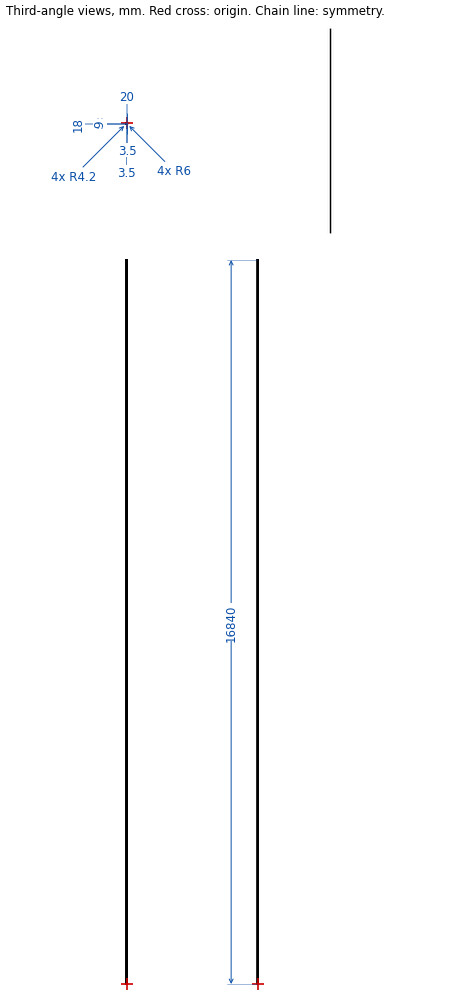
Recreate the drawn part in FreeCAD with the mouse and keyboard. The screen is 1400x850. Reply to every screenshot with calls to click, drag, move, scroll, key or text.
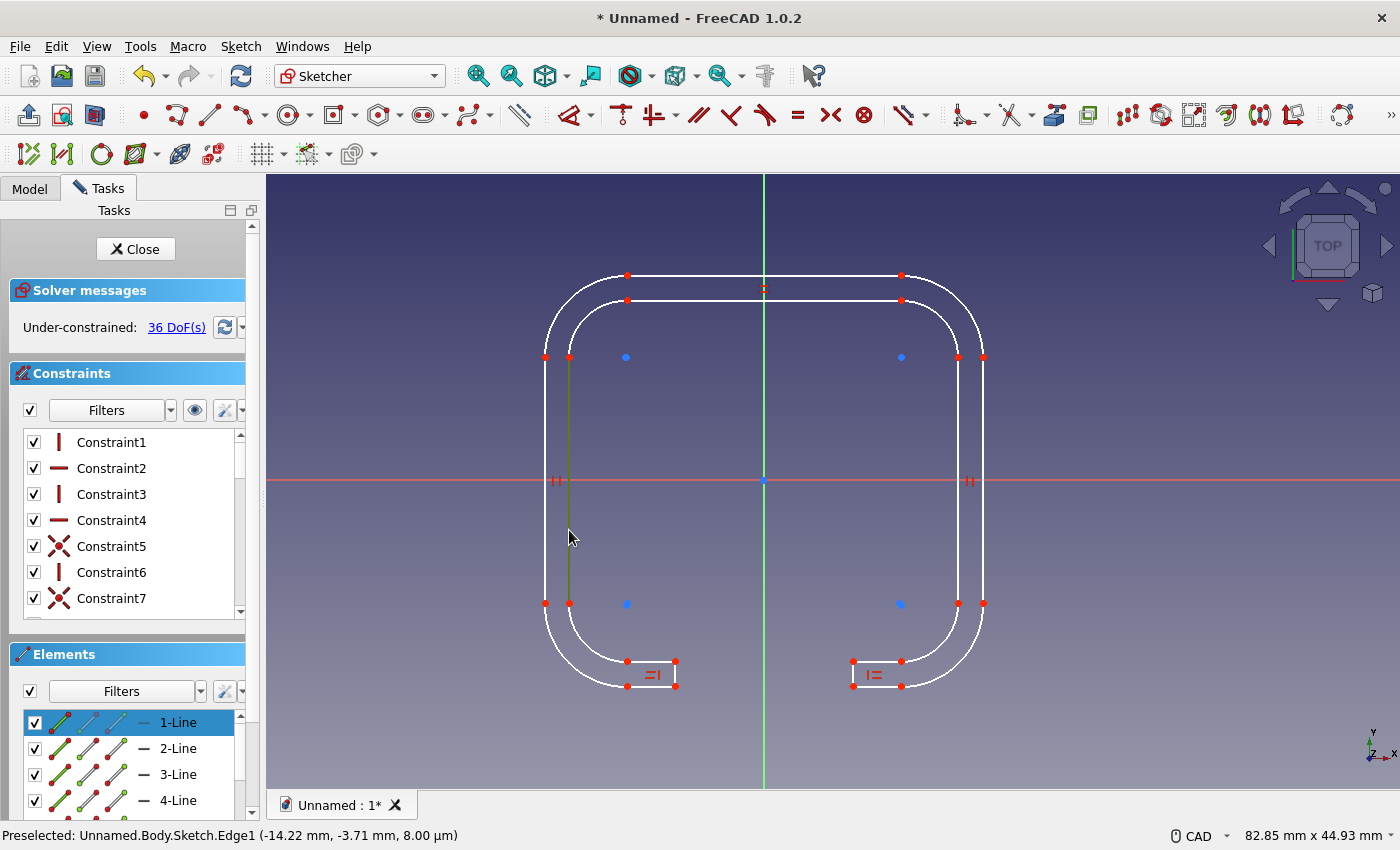
click(601, 307)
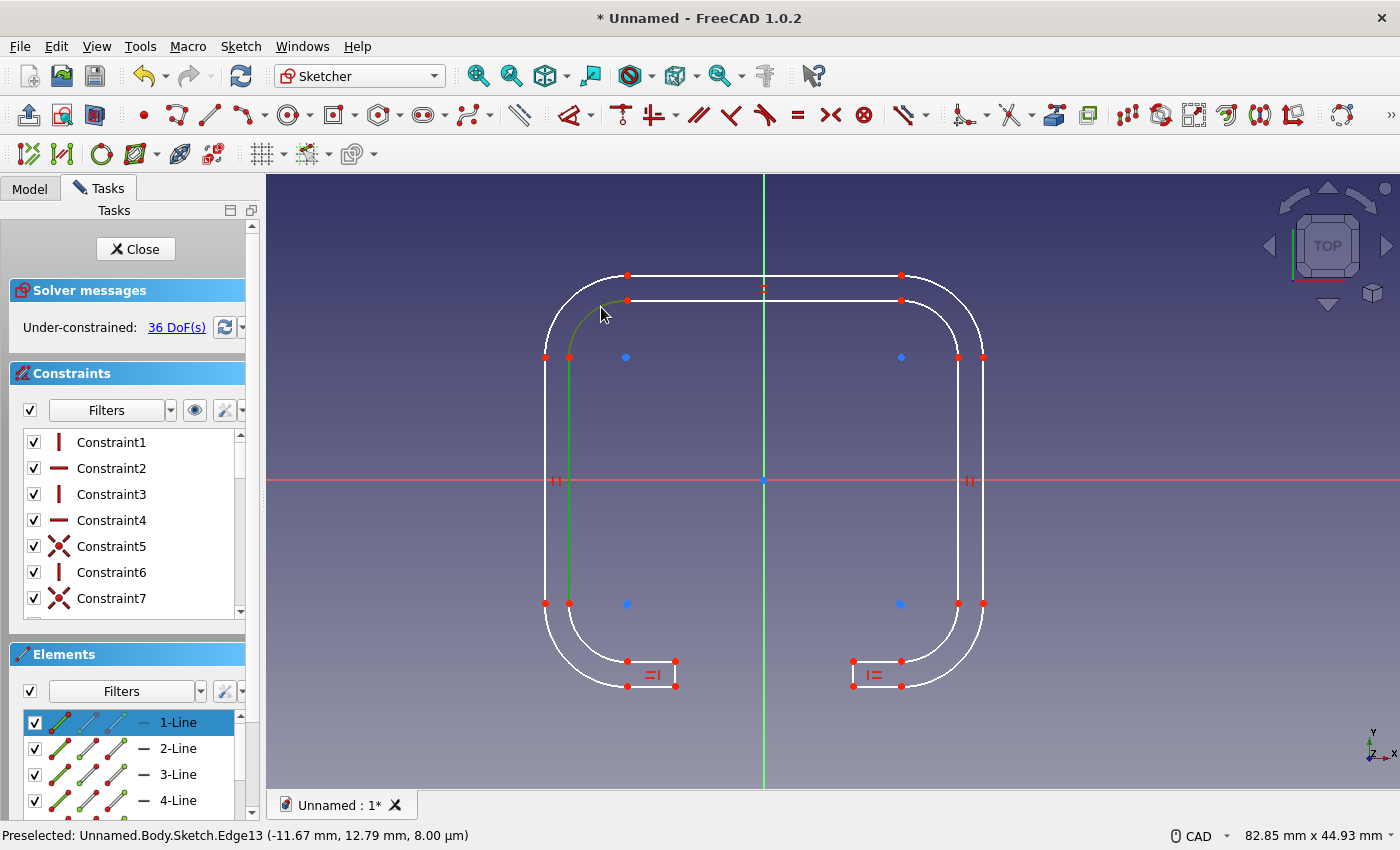
click(765, 116)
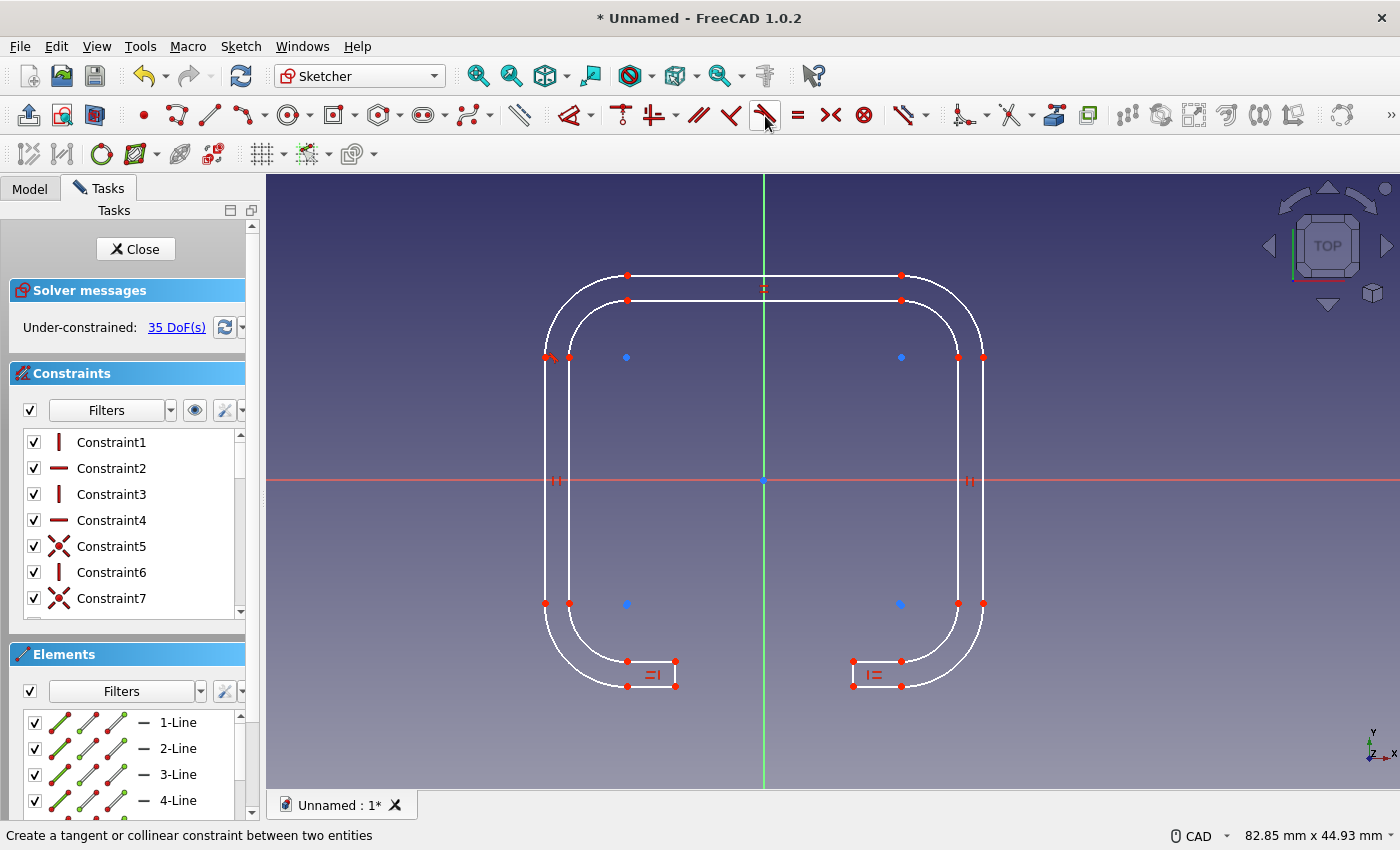
click(569, 530)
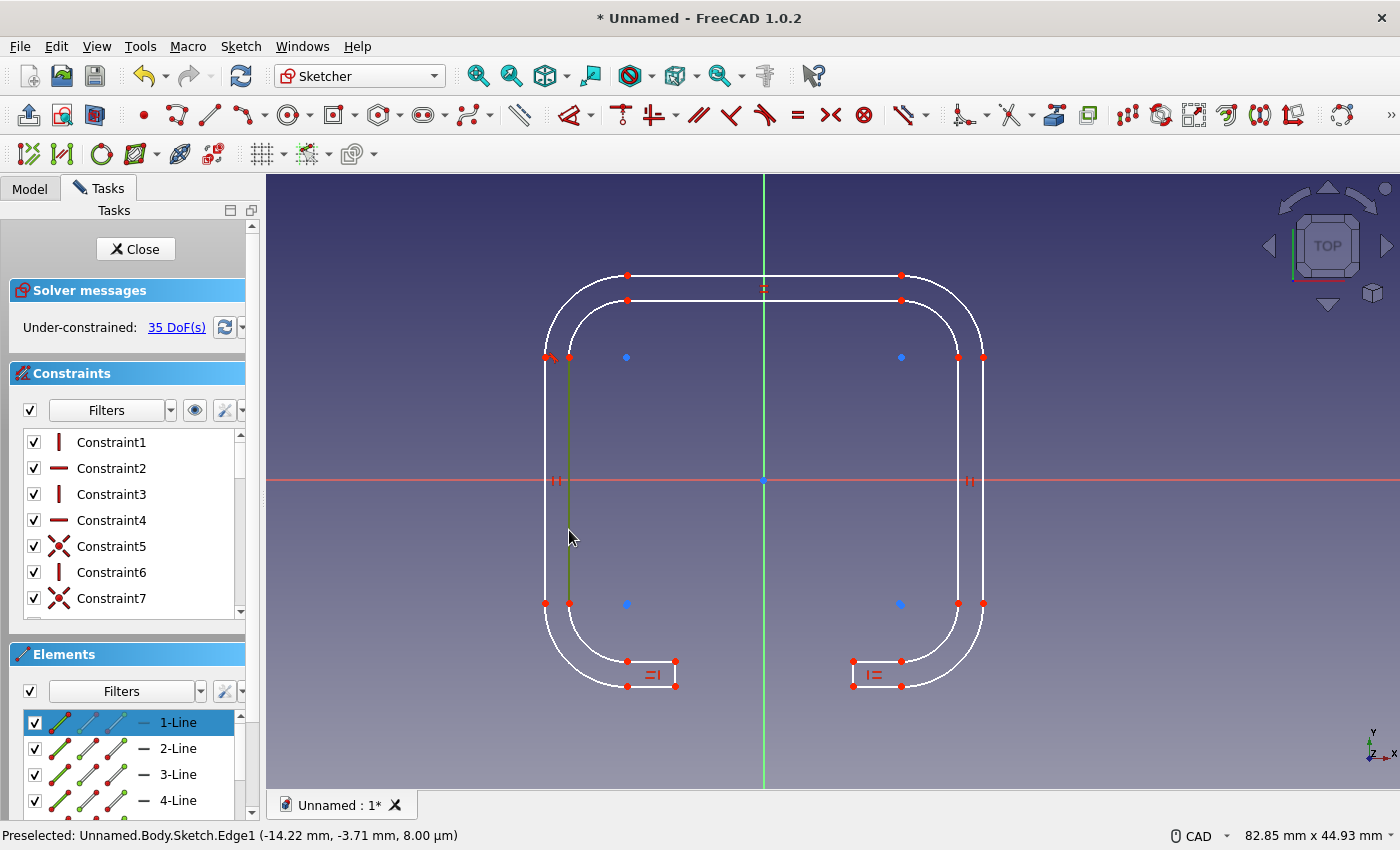
click(575, 630)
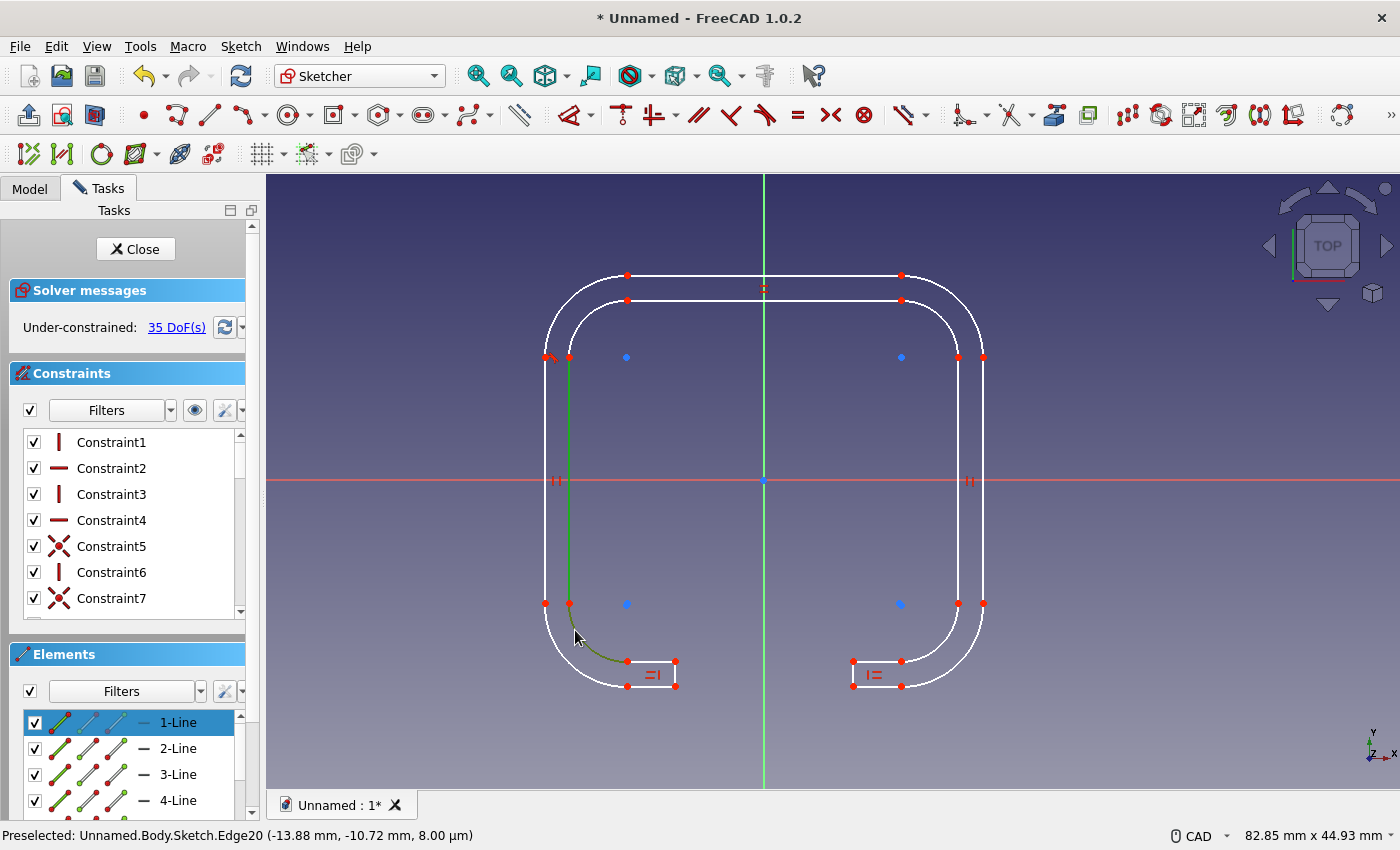
click(765, 116)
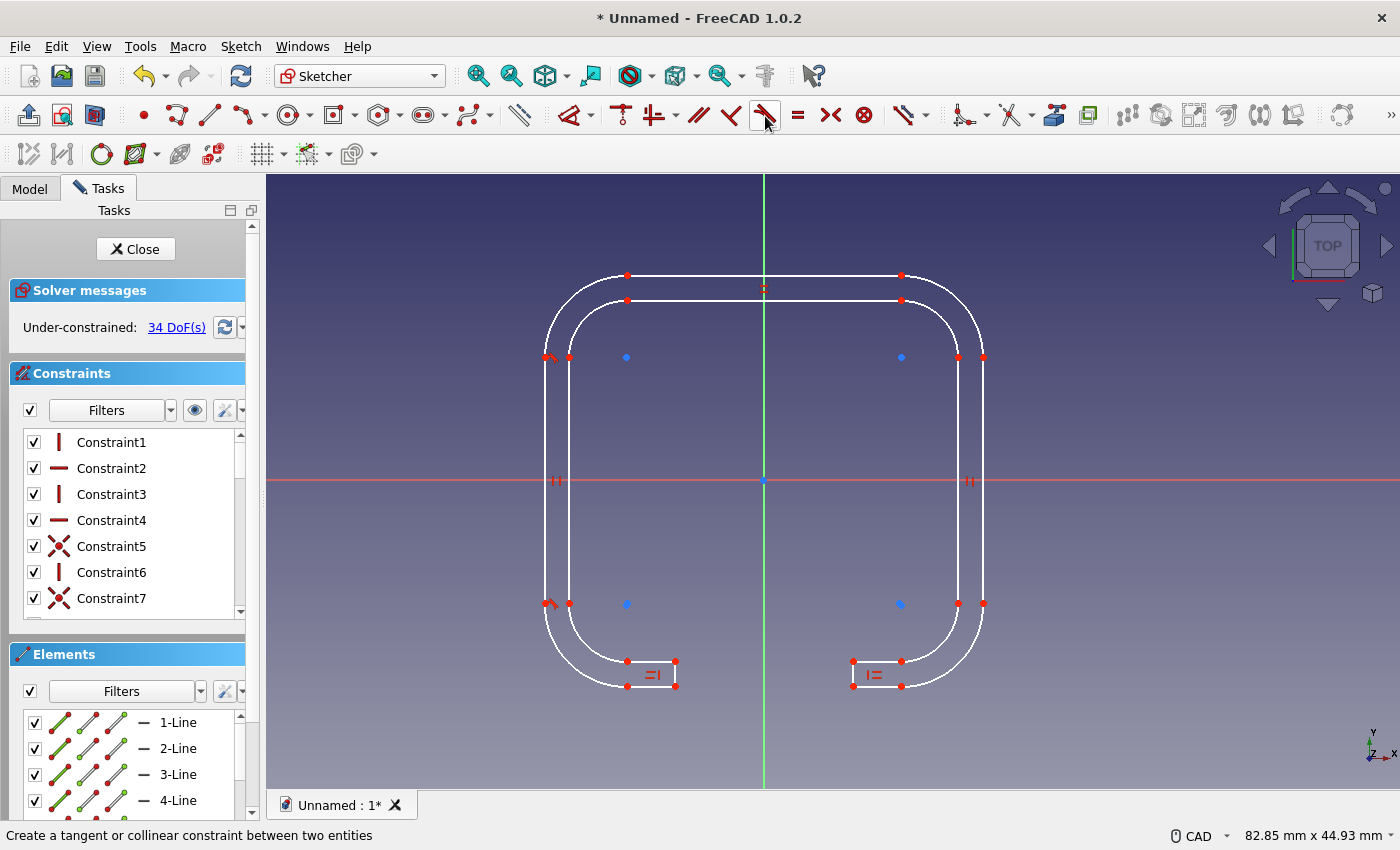
click(709, 301)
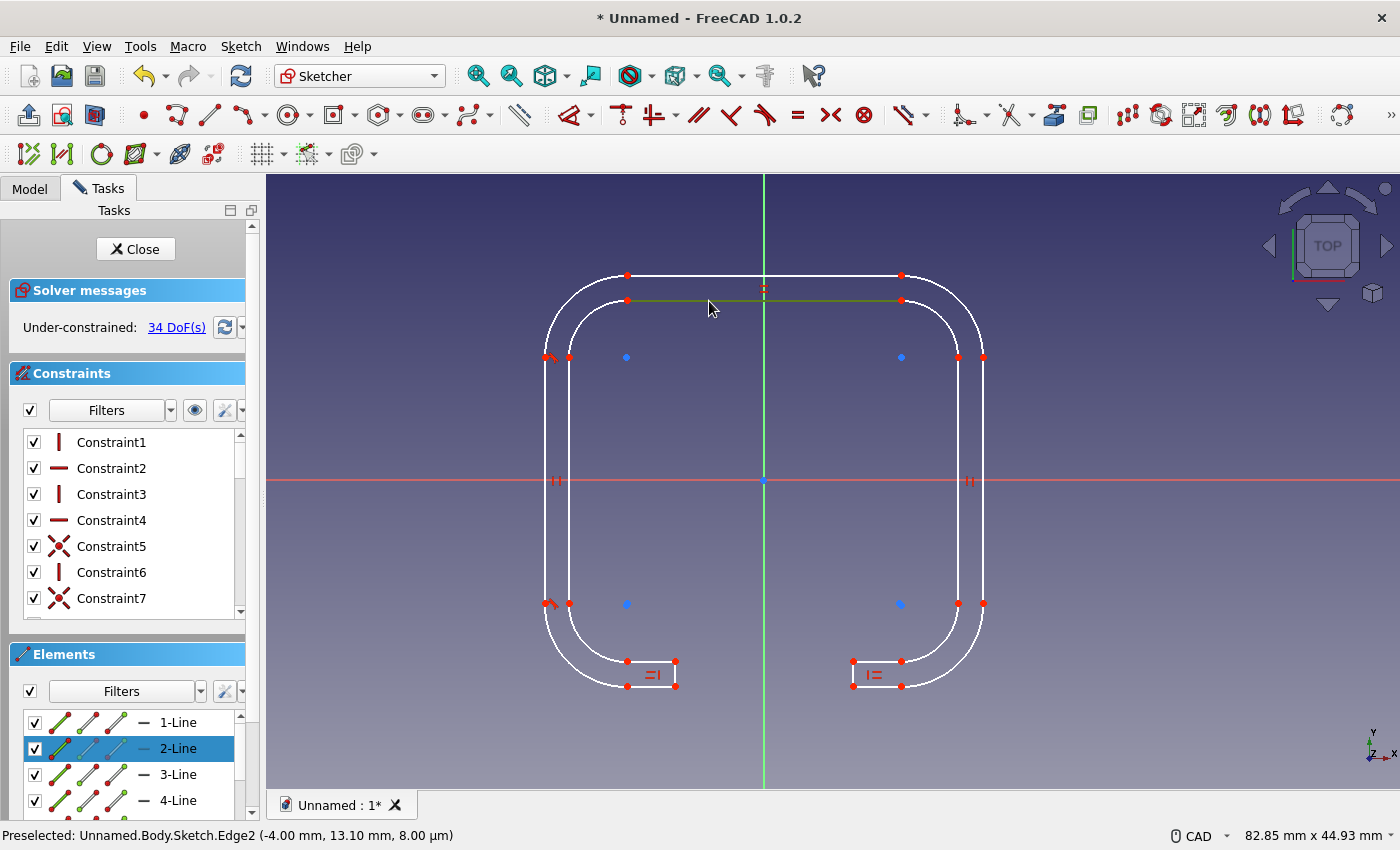
click(601, 307)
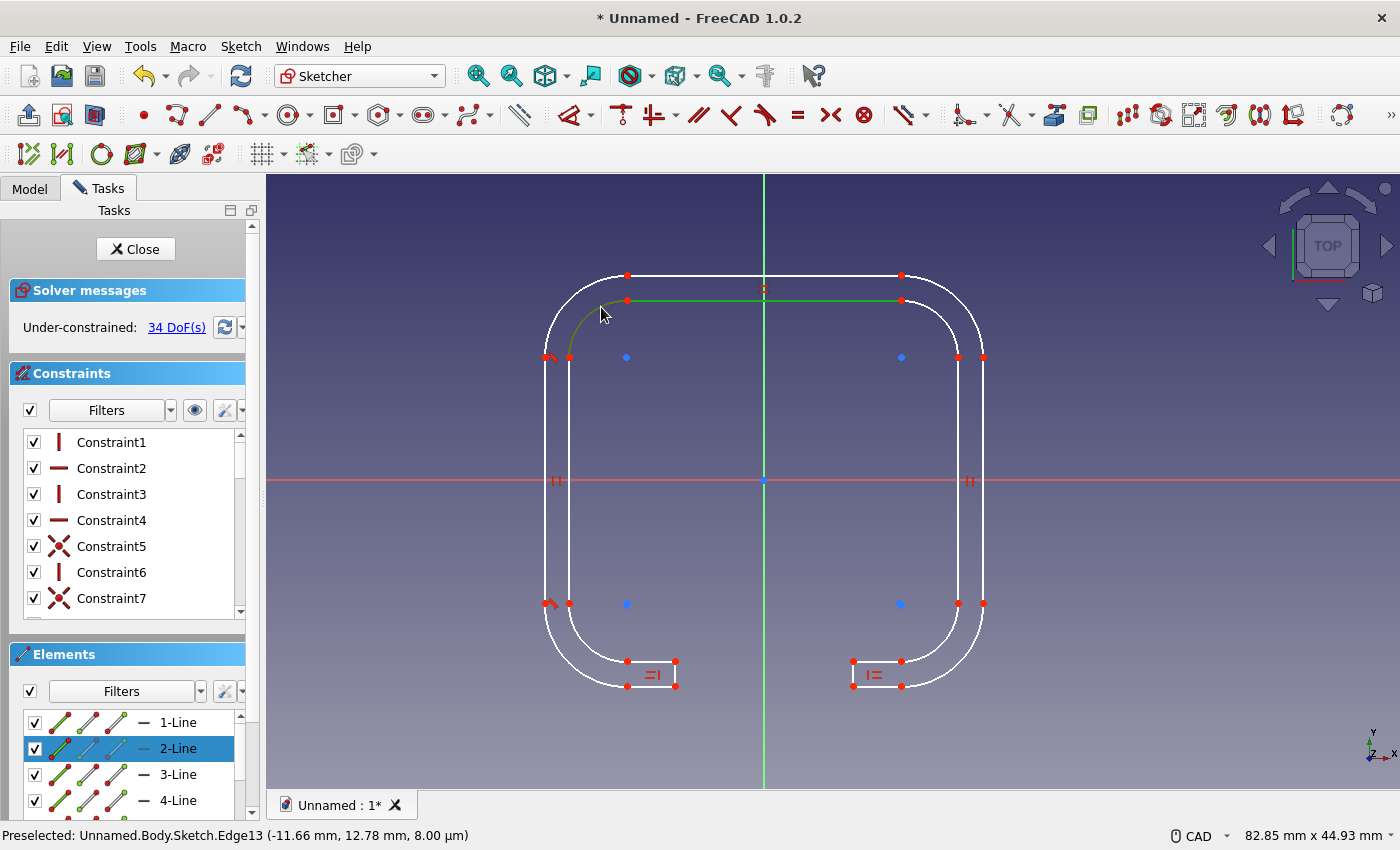
click(765, 116)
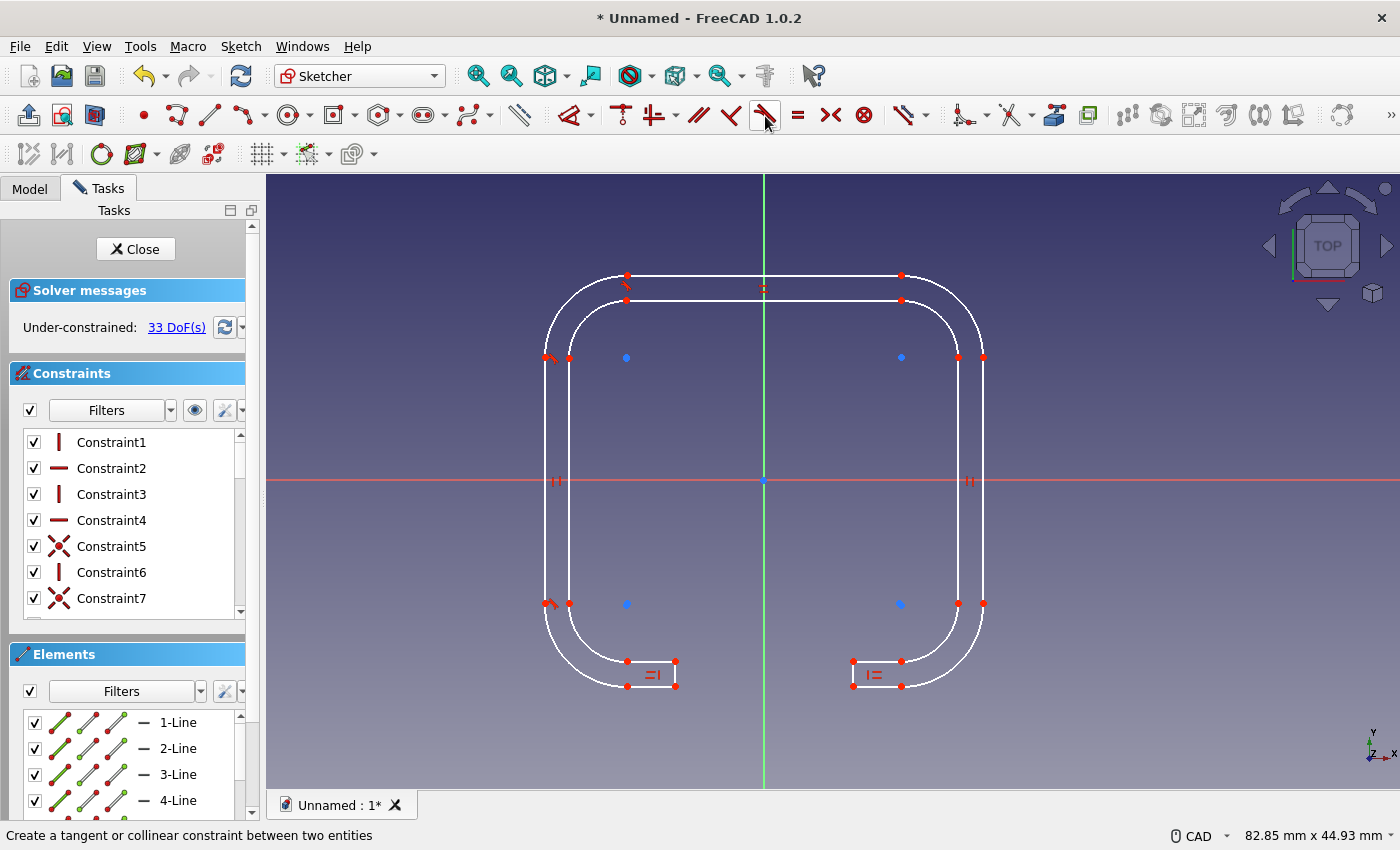
click(709, 301)